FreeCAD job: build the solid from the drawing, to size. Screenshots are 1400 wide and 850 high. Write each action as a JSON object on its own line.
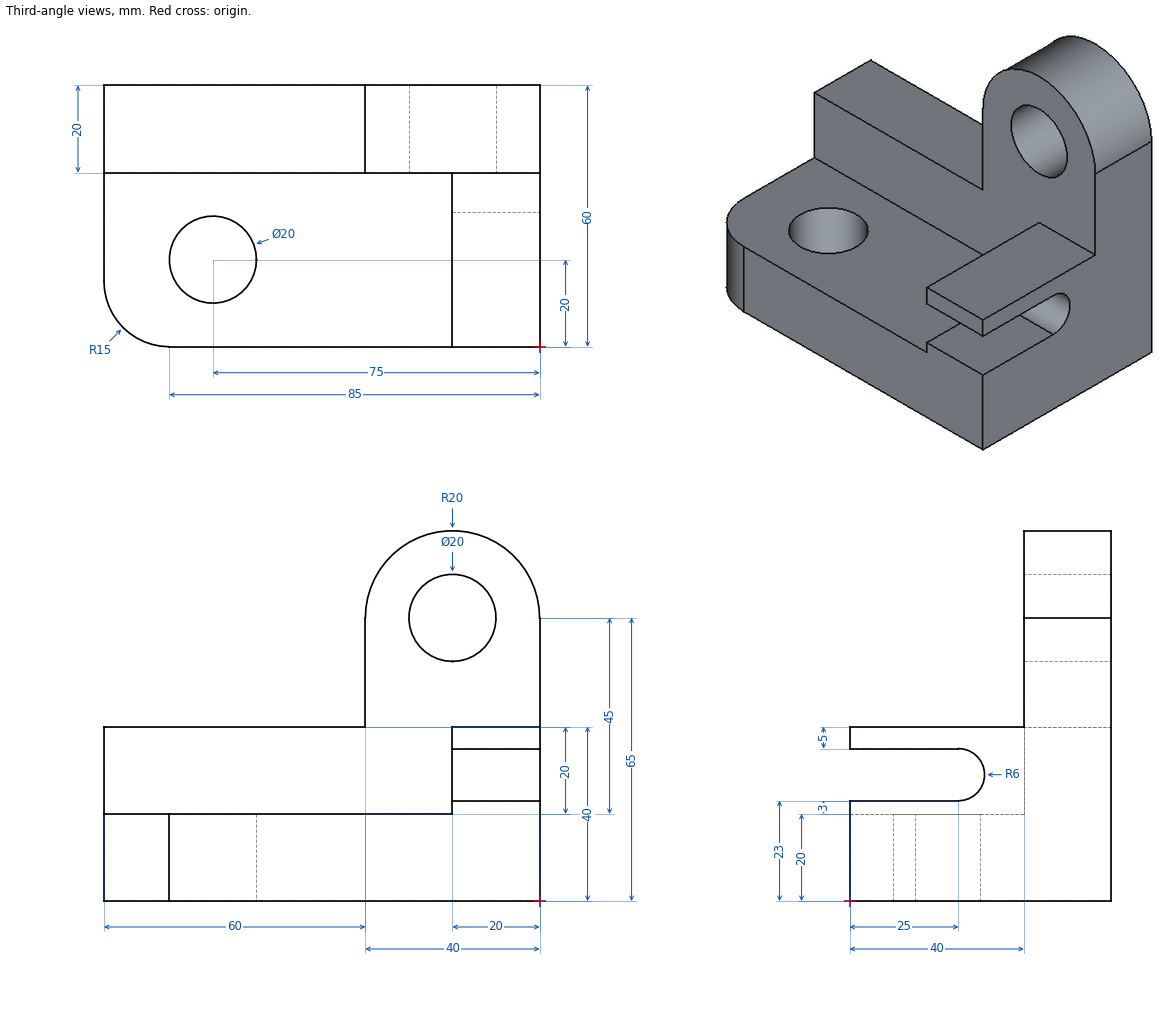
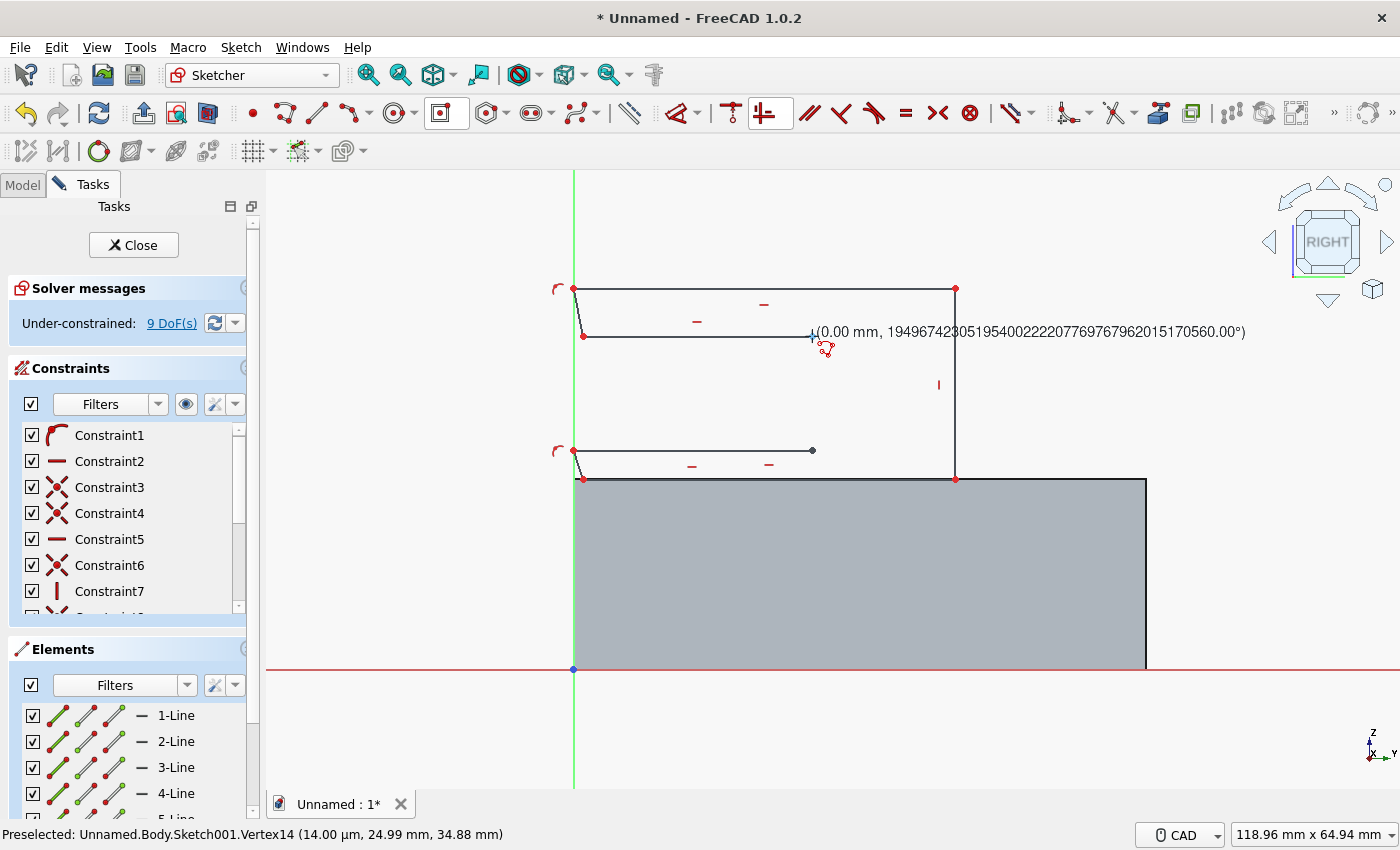
{"action": "left_click", "coordinate": [350, 114]}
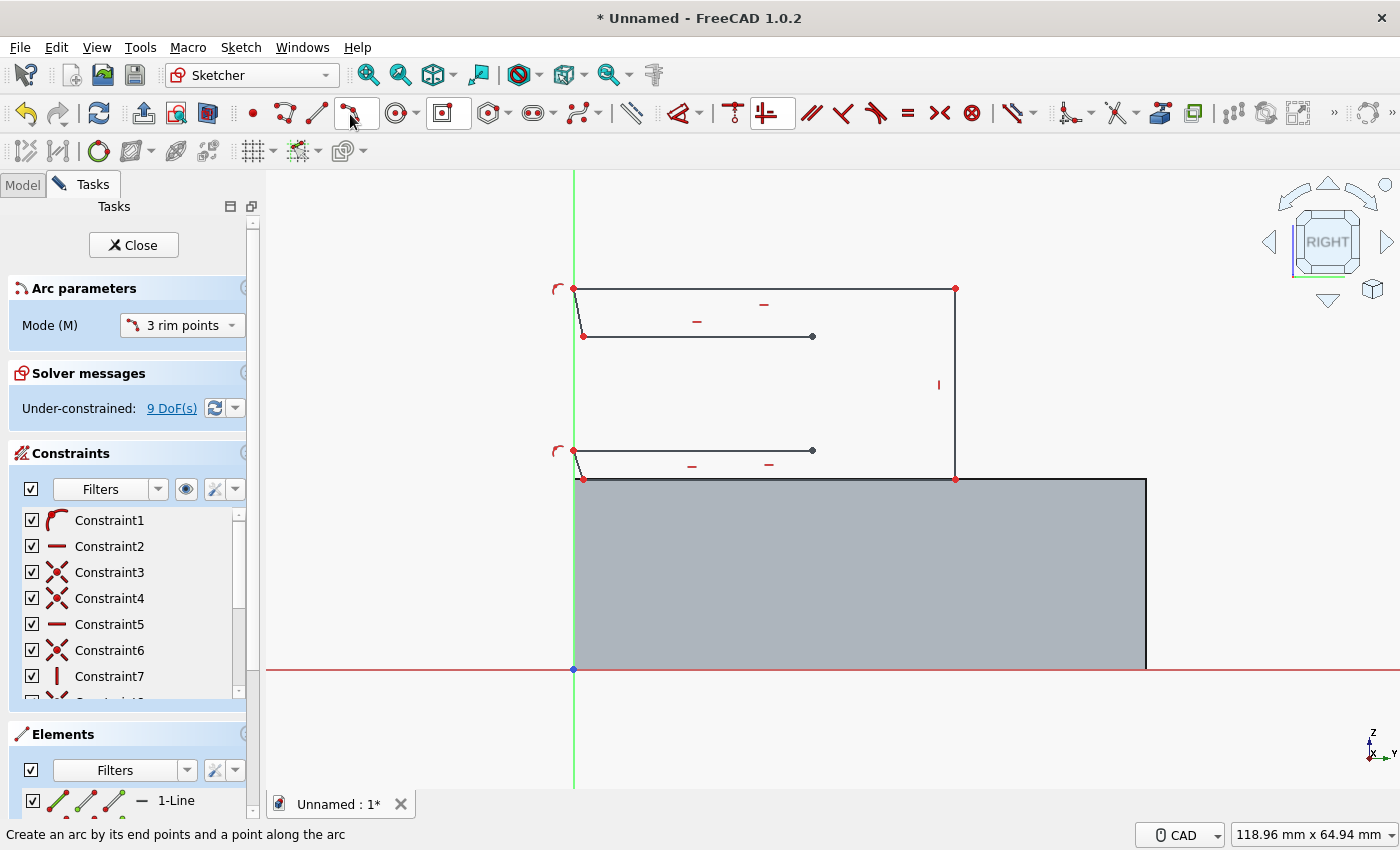
{"action": "left_click", "coordinate": [812, 337]}
{"action": "left_click", "coordinate": [812, 451]}
{"action": "left_click", "coordinate": [869, 393]}
{"action": "key", "text": "Escape"}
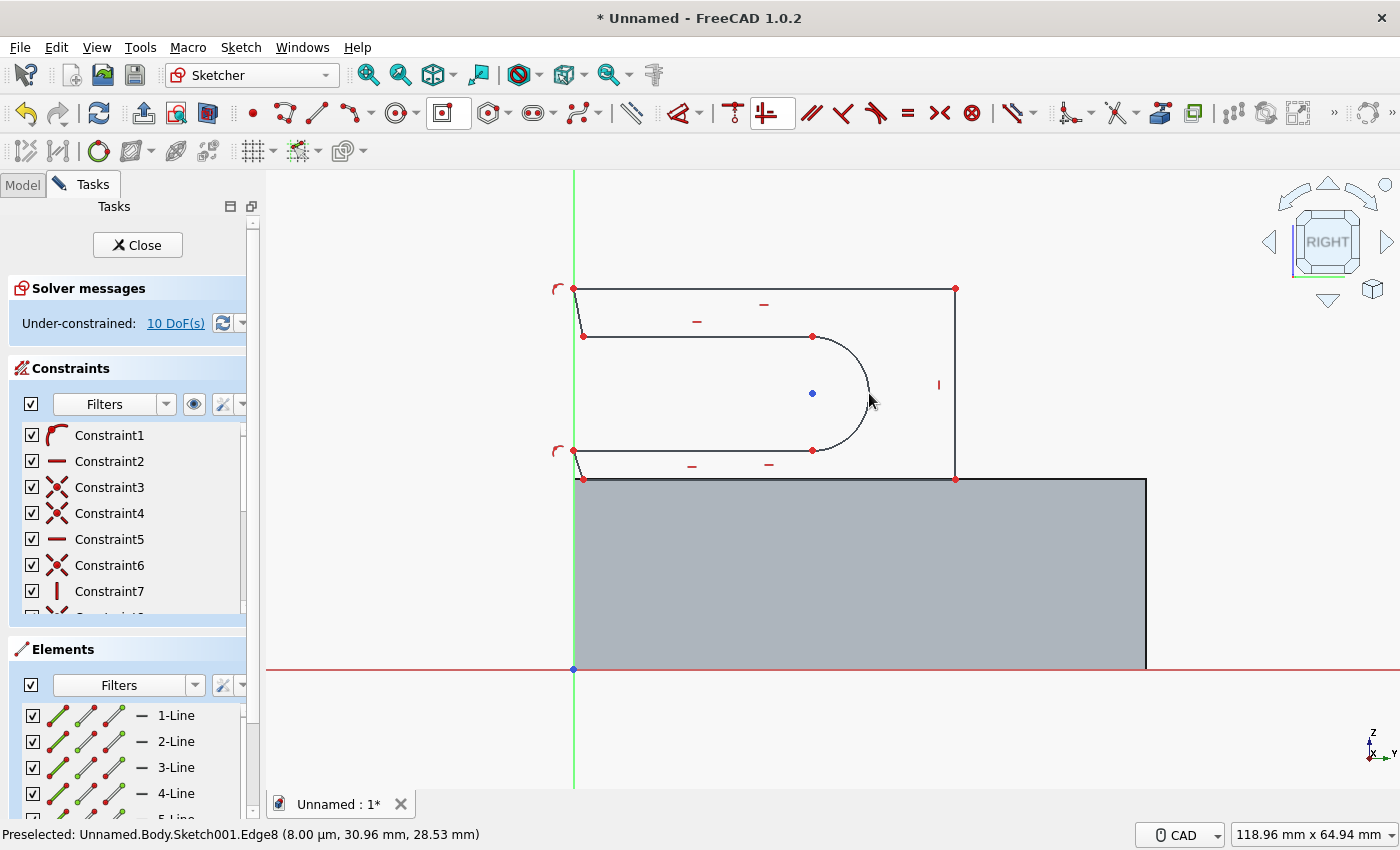
{"action": "left_click", "coordinate": [741, 451]}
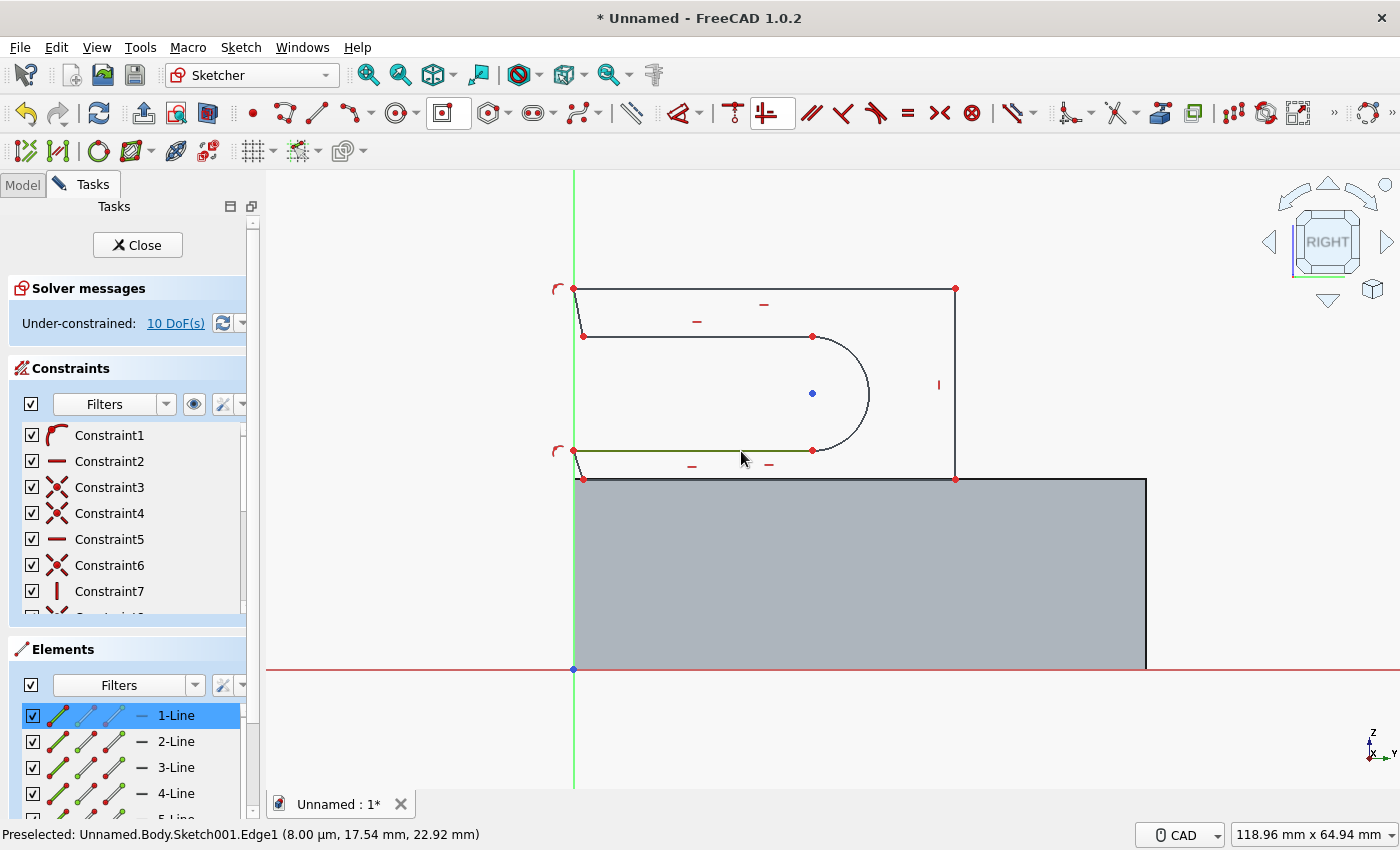
{"action": "left_click", "coordinate": [858, 428]}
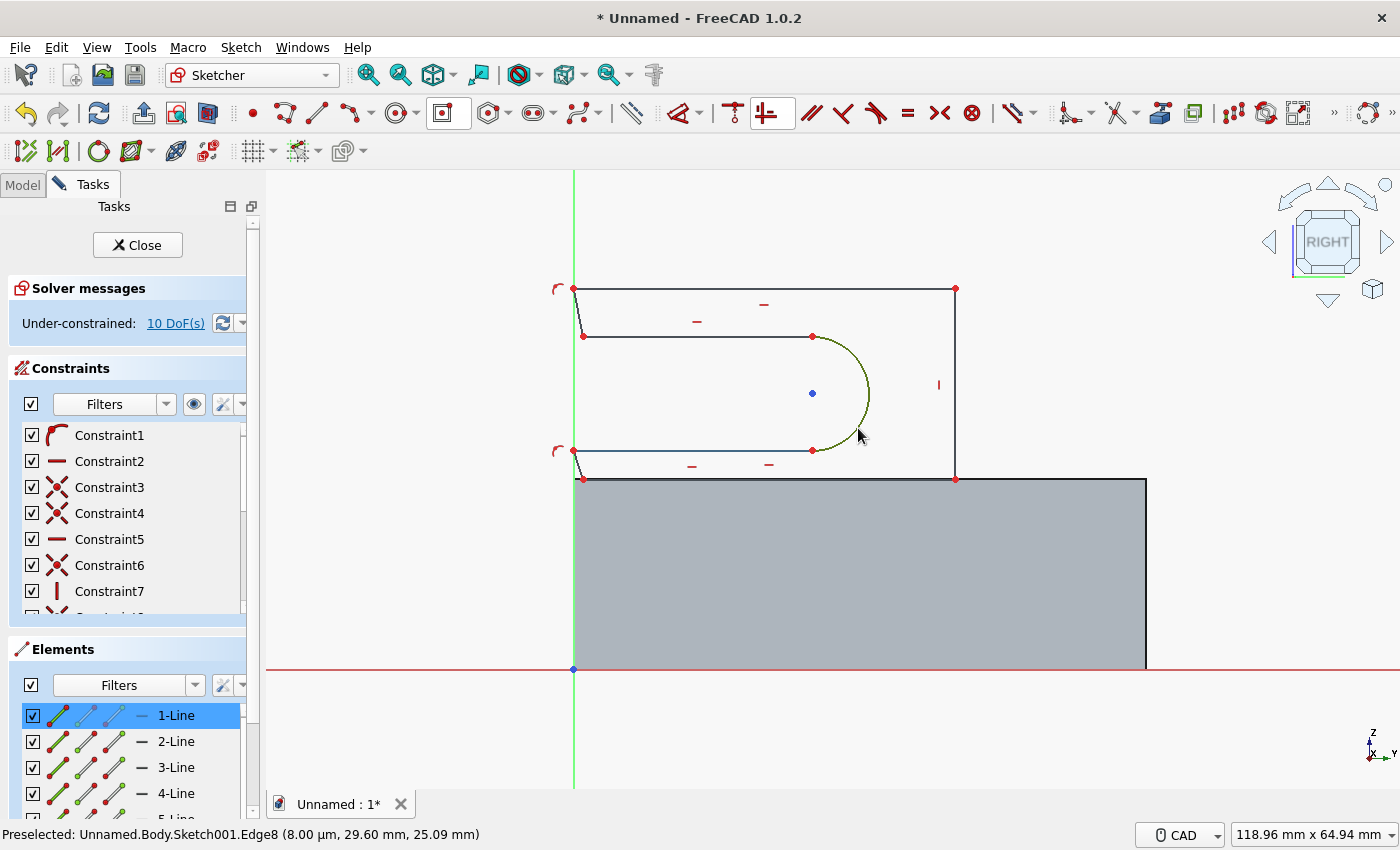
{"action": "key", "text": "t"}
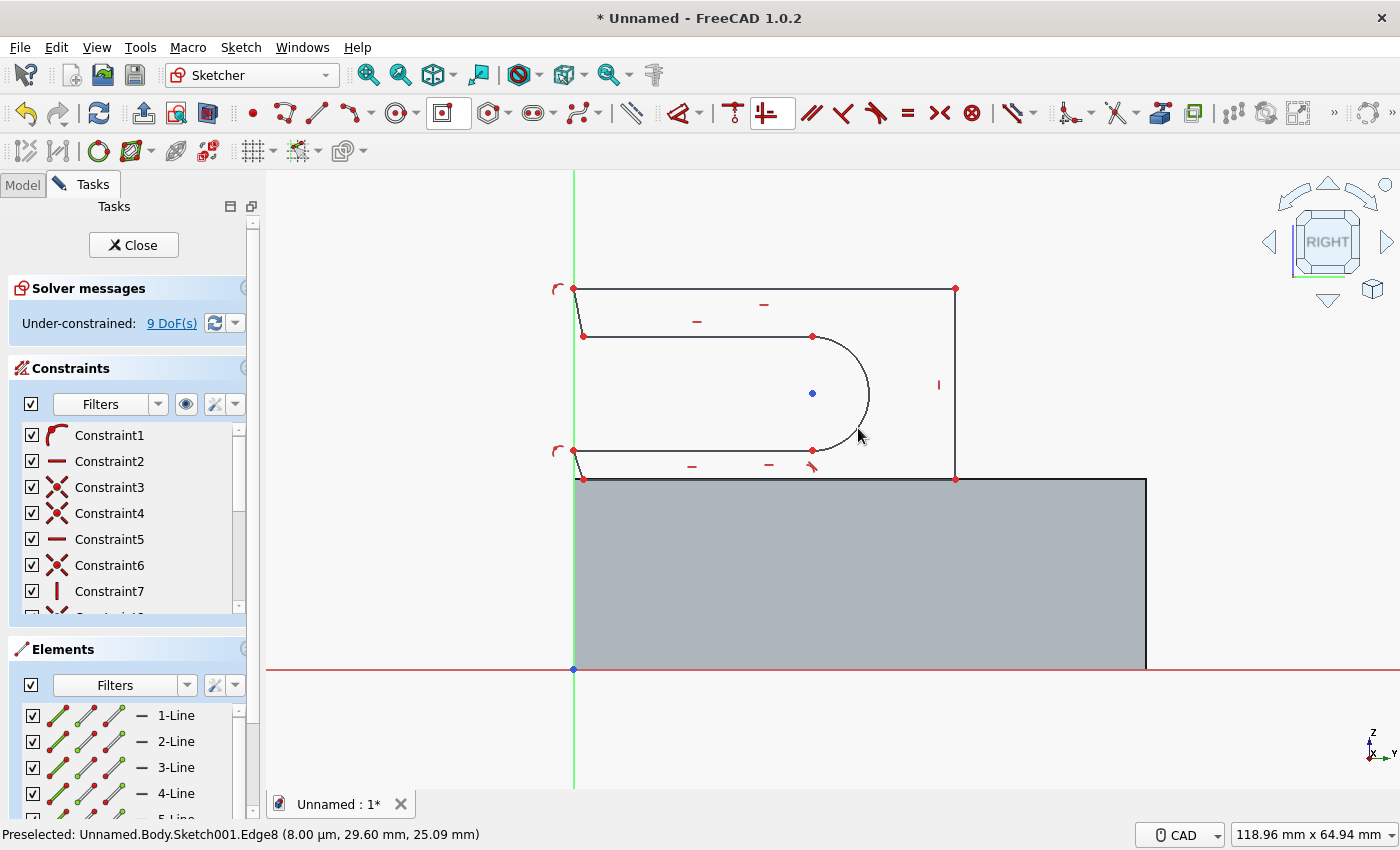
{"action": "left_click", "coordinate": [652, 337]}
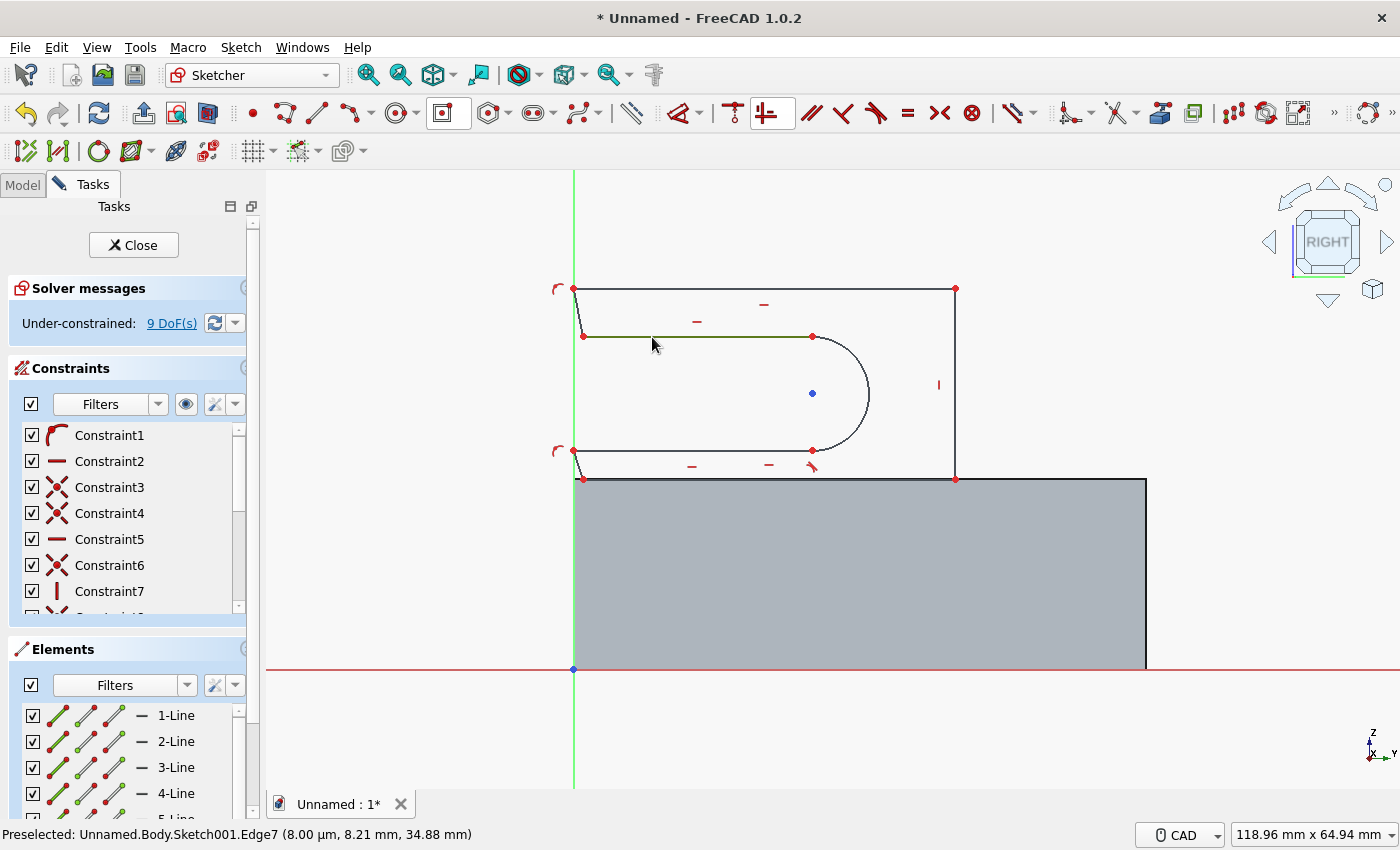
{"action": "left_click", "coordinate": [858, 428]}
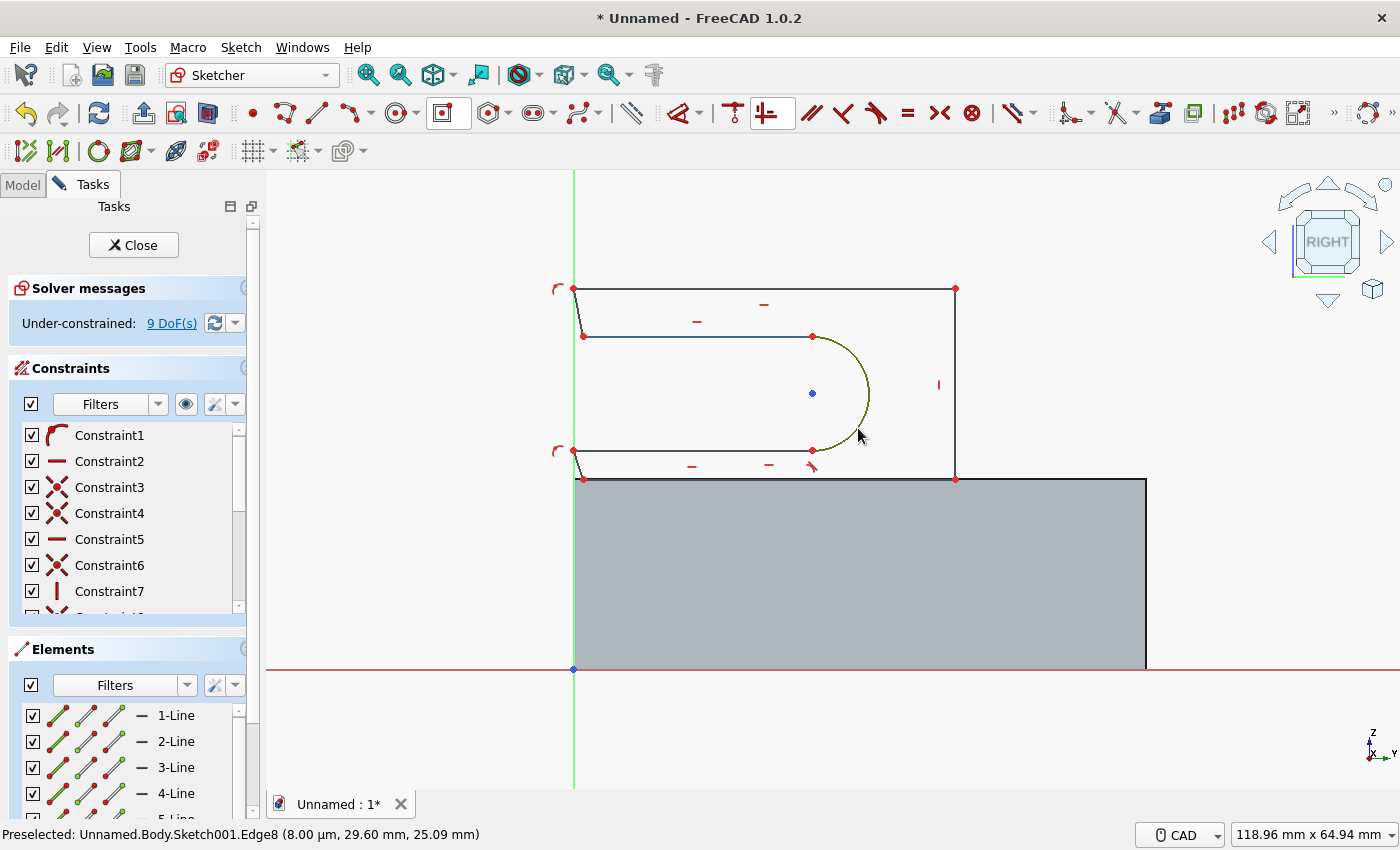
{"action": "key", "text": "t"}